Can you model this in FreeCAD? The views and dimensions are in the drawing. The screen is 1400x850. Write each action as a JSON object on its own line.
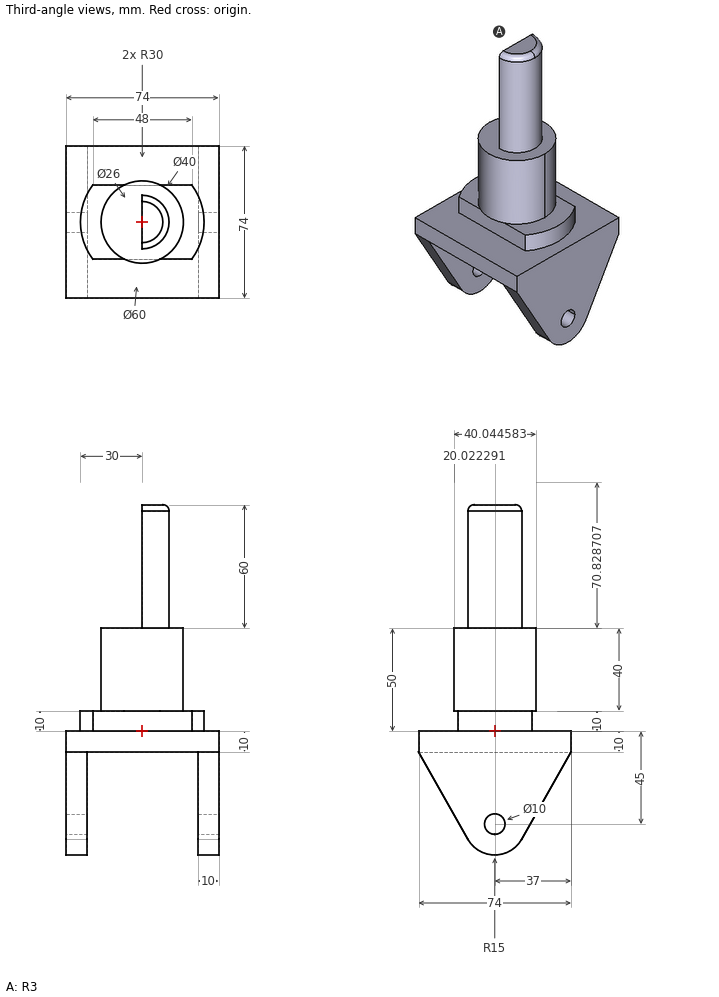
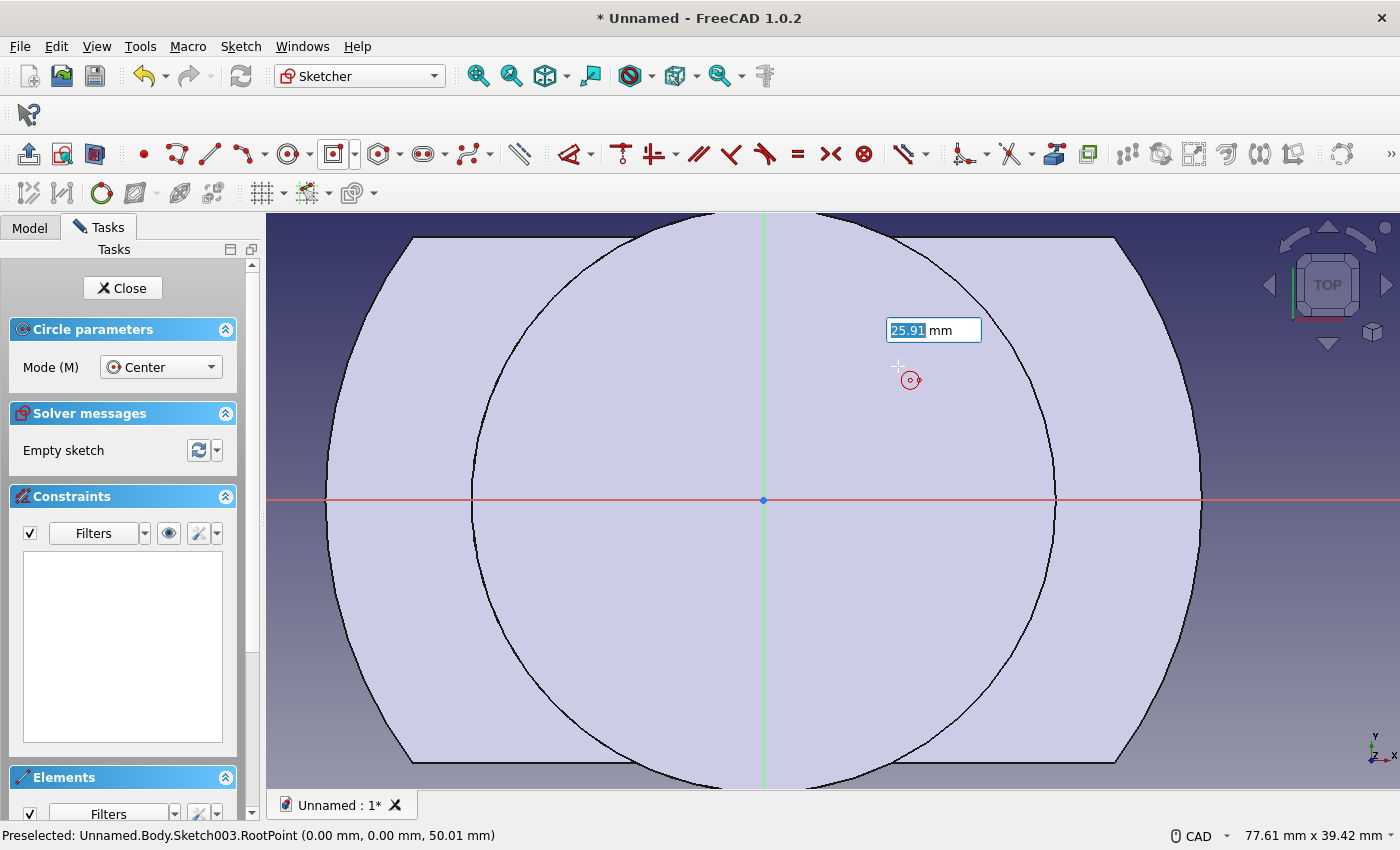
{"action": "type", "text": "26"}
{"action": "key", "text": "Return"}
{"action": "key", "text": "Escape"}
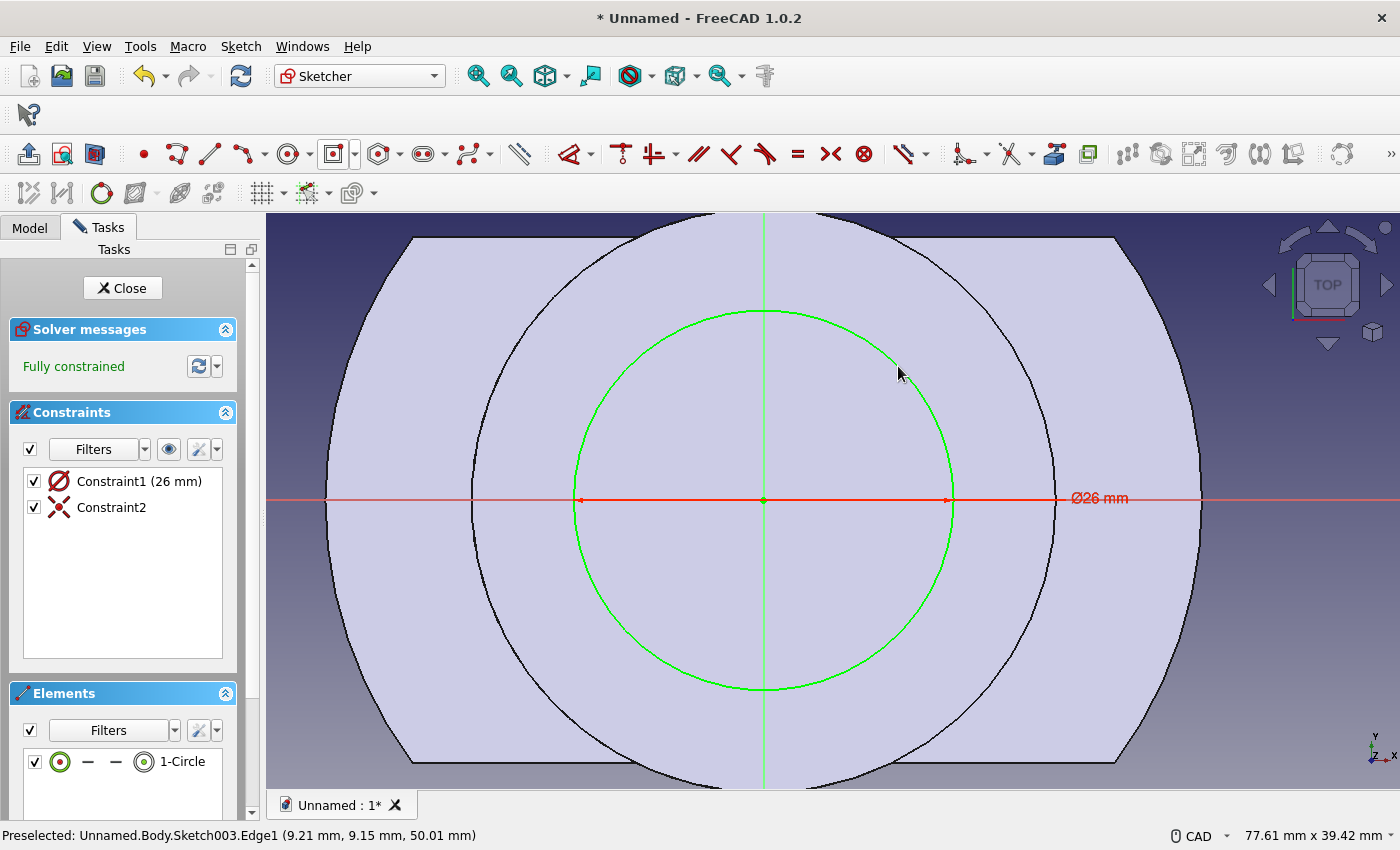
{"action": "left_click", "coordinate": [123, 288]}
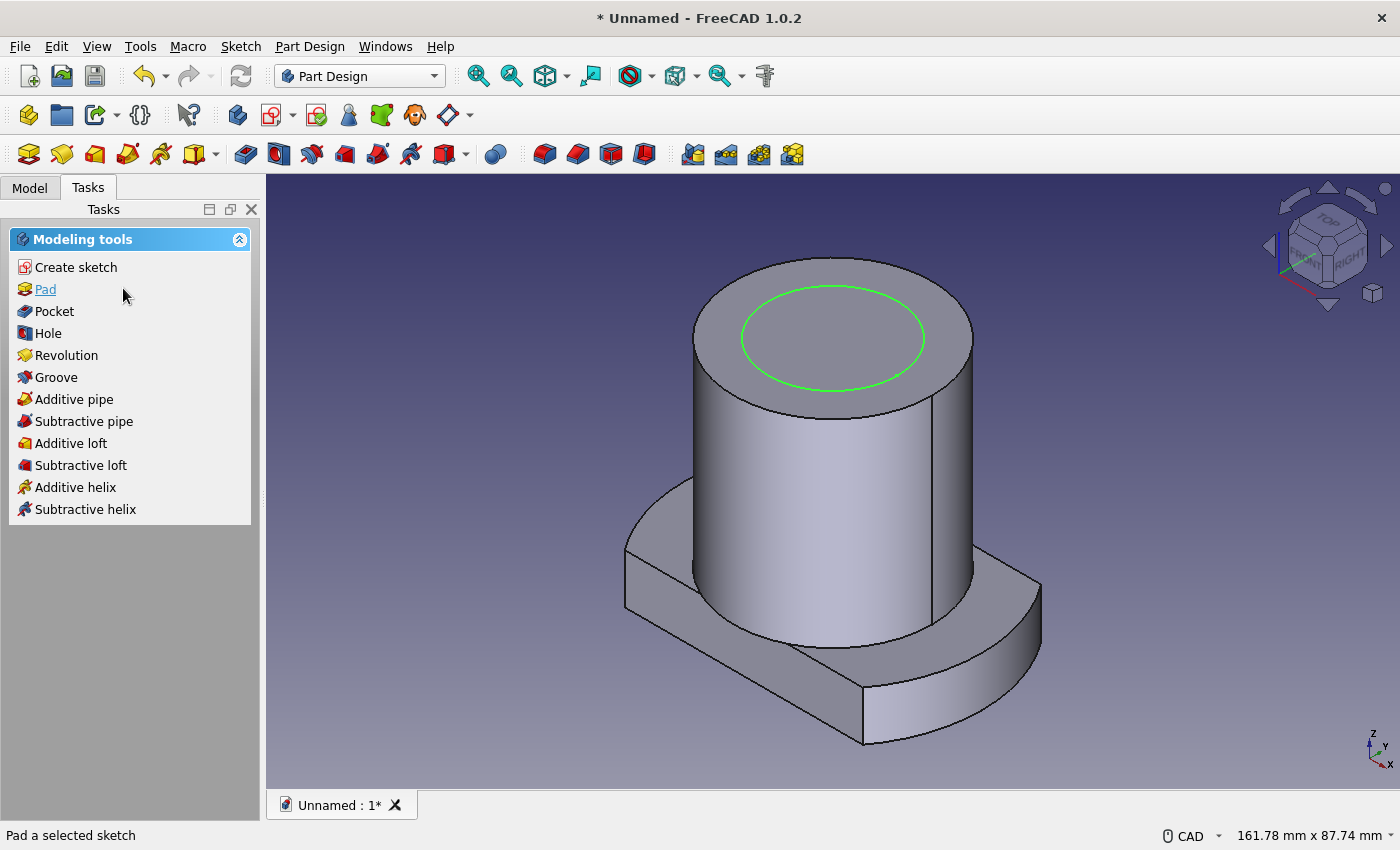
{"action": "left_click", "coordinate": [29, 154]}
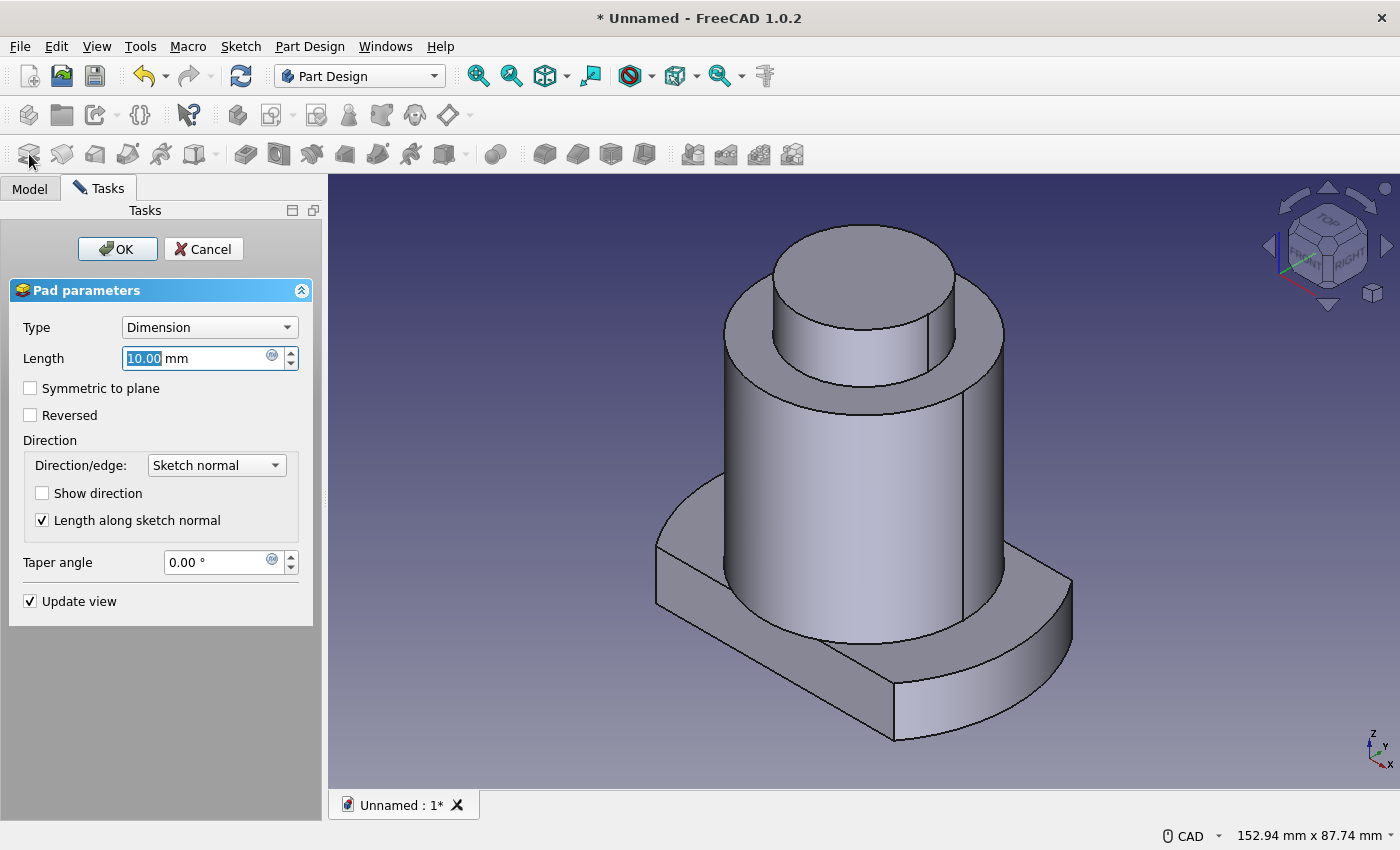
{"action": "type", "text": "60"}
{"action": "key", "text": "Tab"}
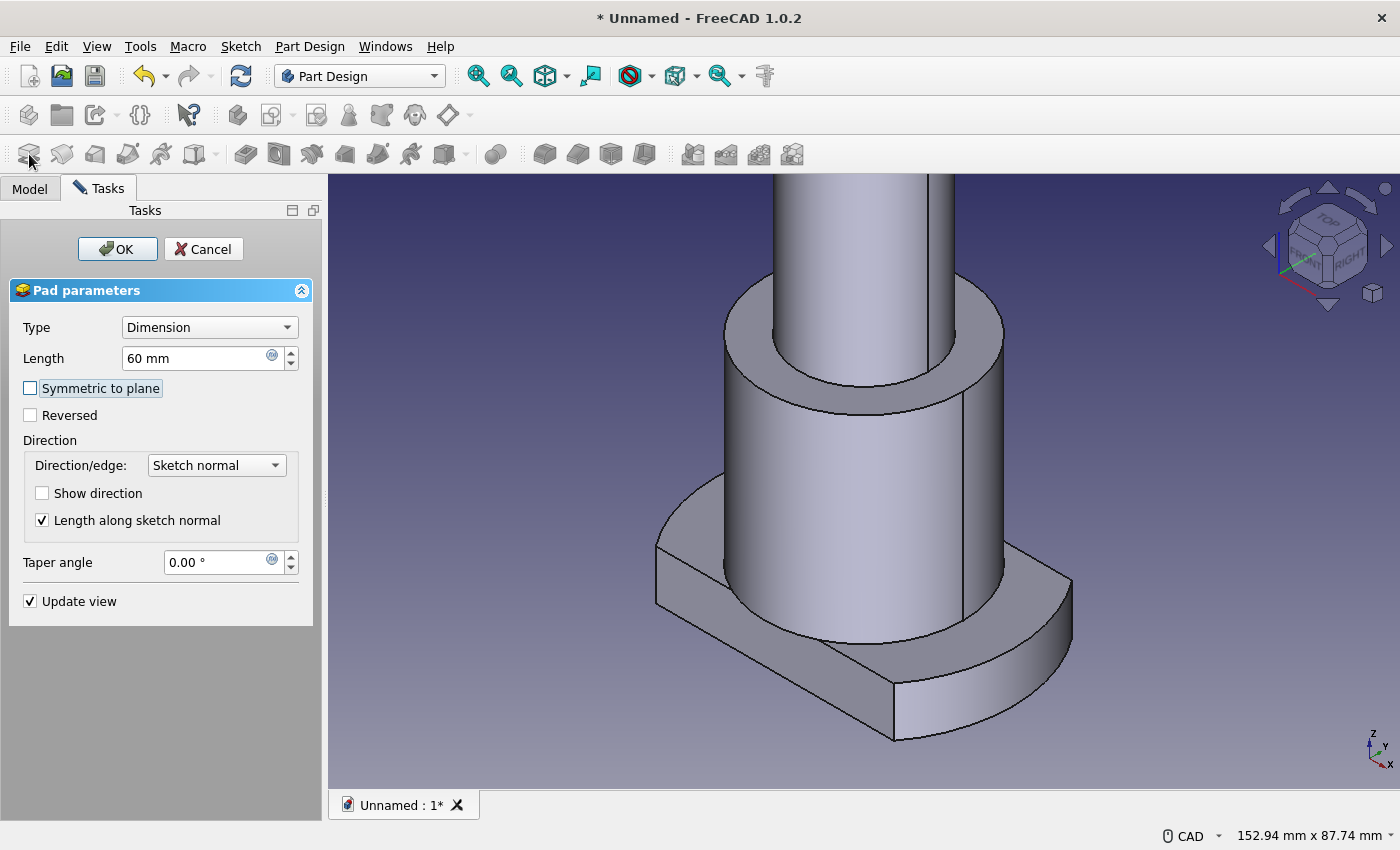
{"action": "left_click", "coordinate": [118, 249]}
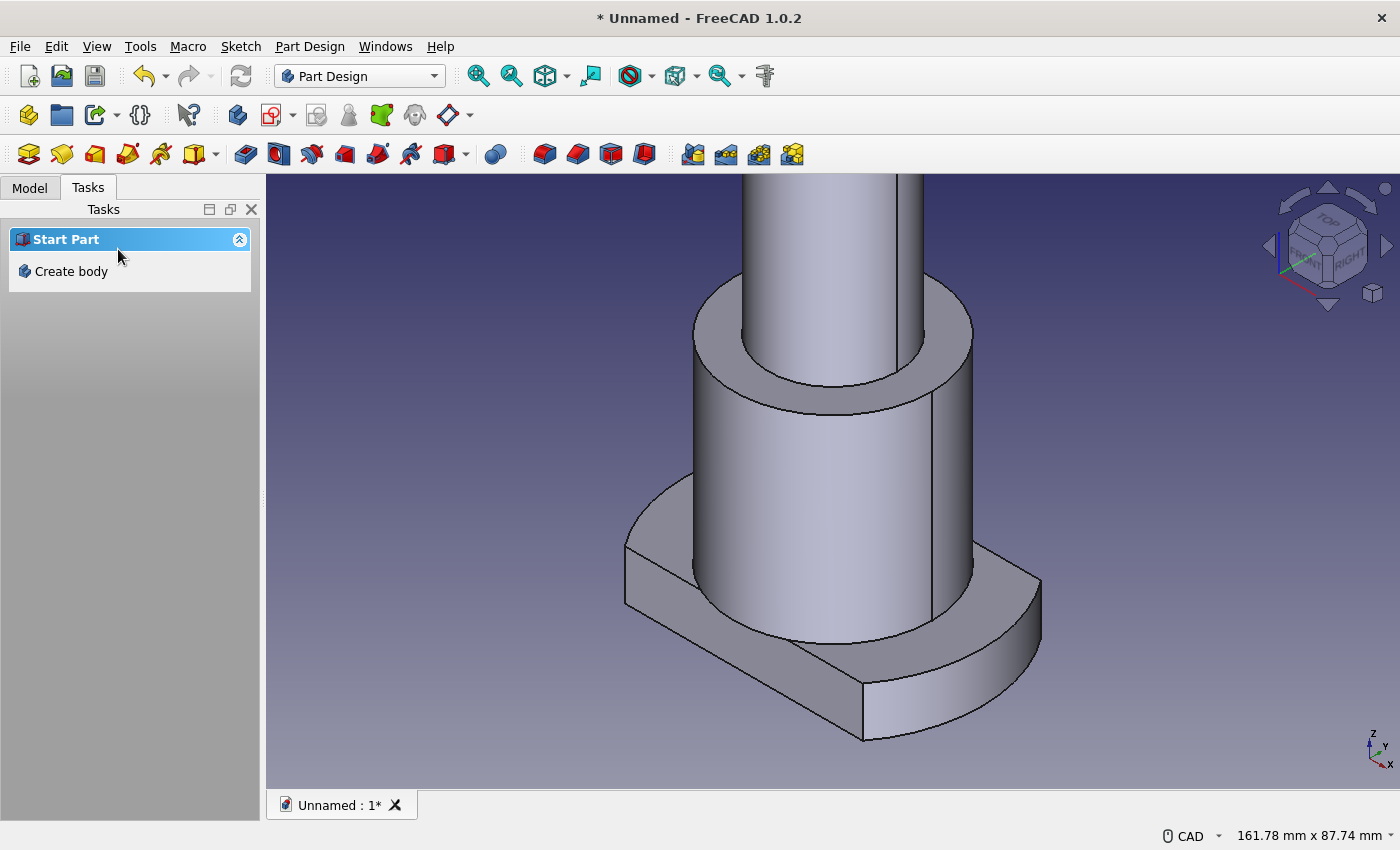
{"action": "left_click", "coordinate": [479, 76]}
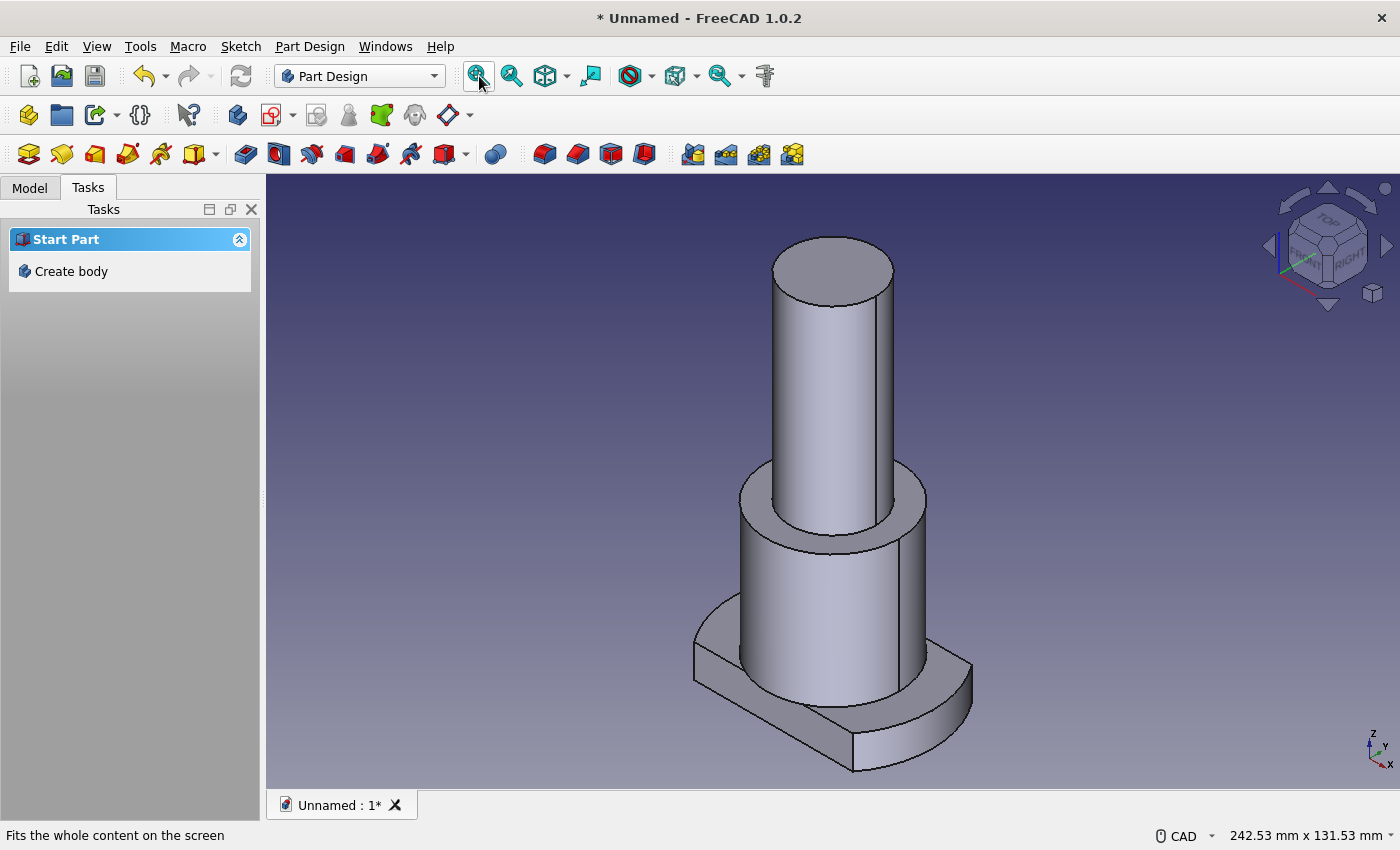
{"action": "left_click", "coordinate": [861, 239]}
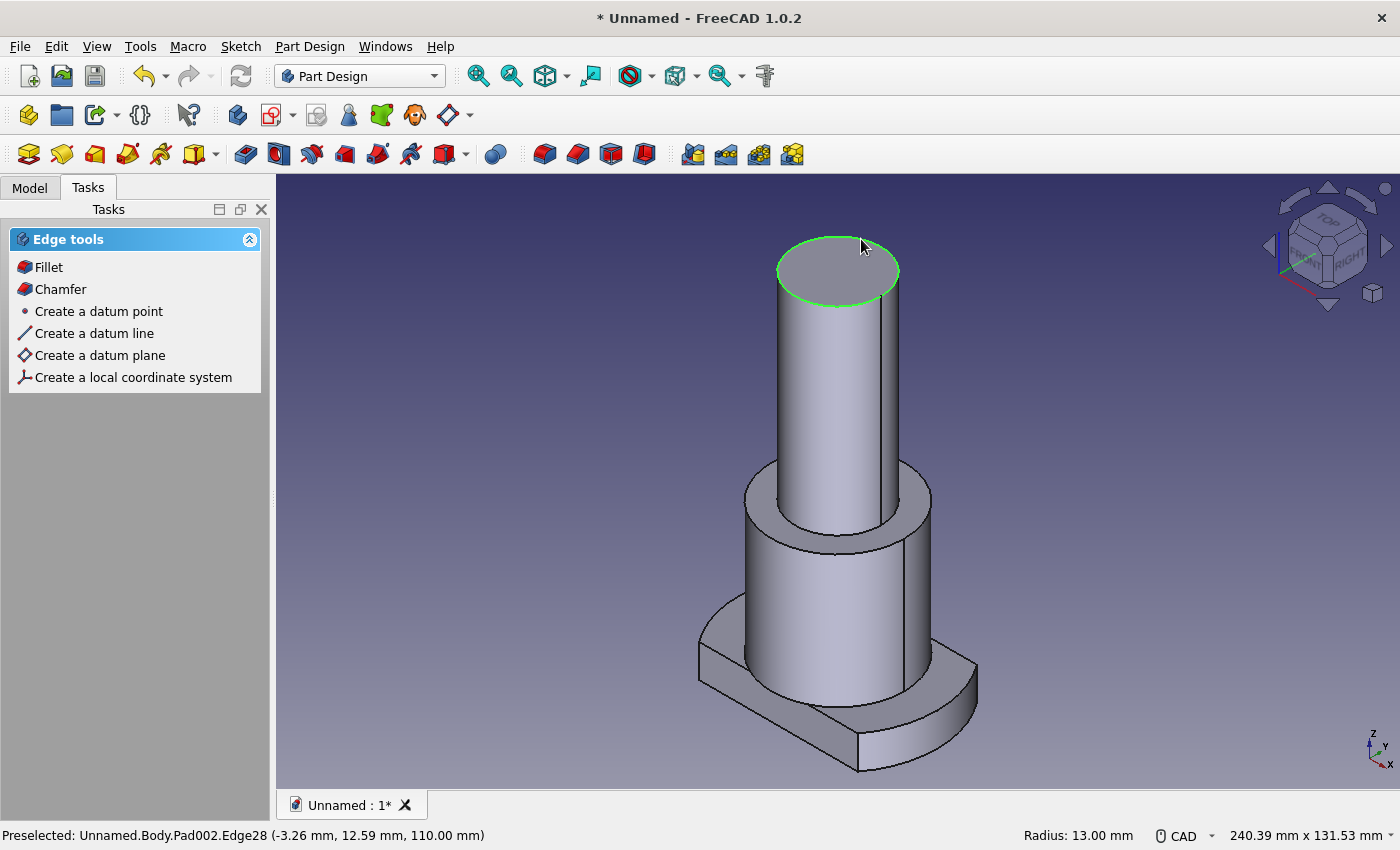
{"action": "left_click", "coordinate": [545, 154]}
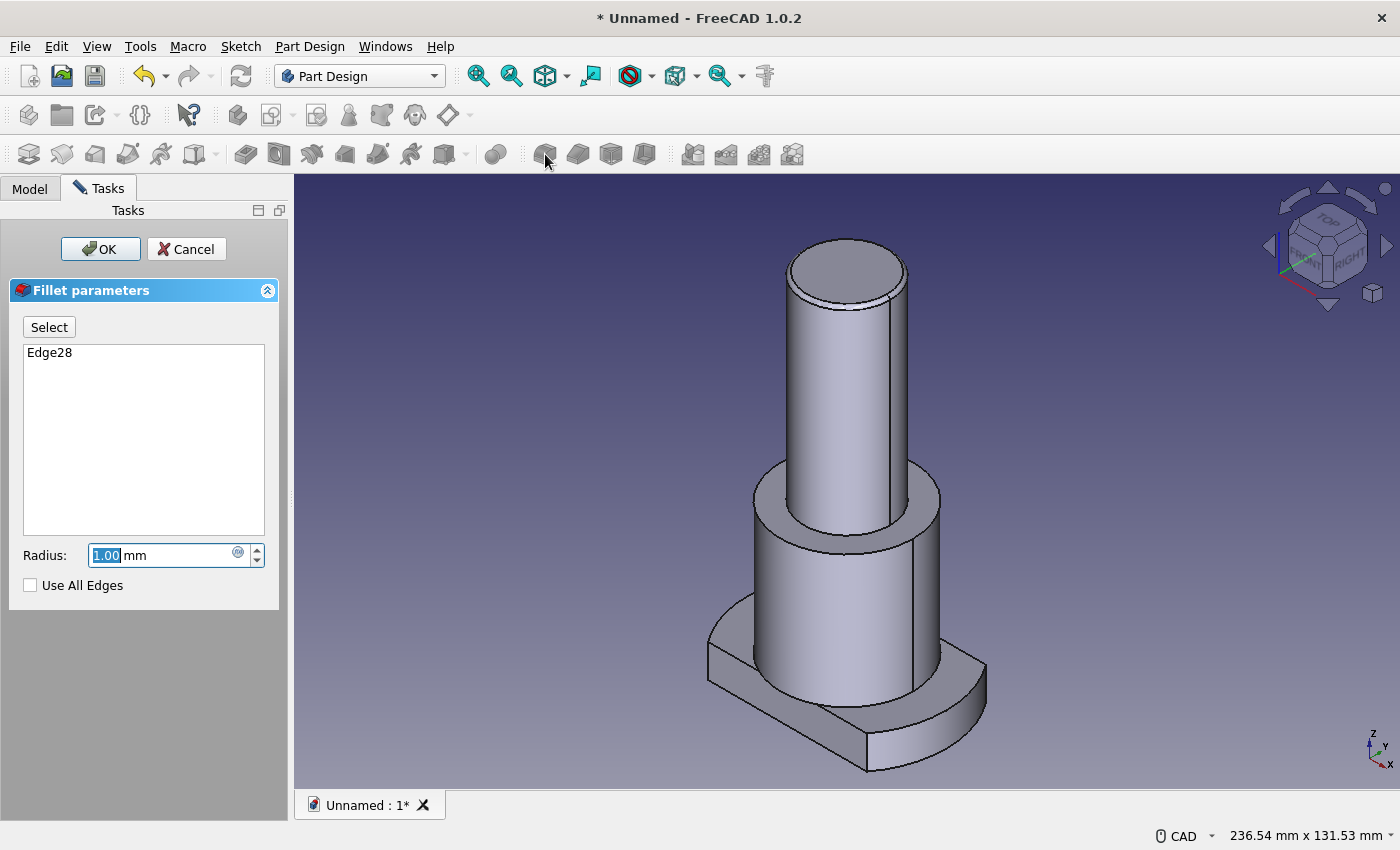
{"action": "type", "text": "3"}
{"action": "key", "text": "Tab"}